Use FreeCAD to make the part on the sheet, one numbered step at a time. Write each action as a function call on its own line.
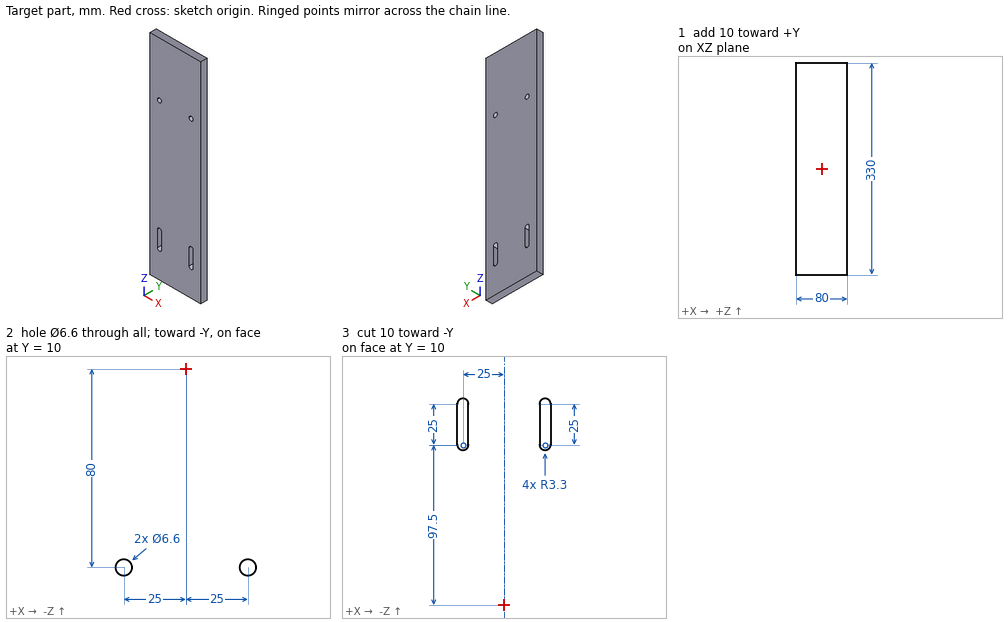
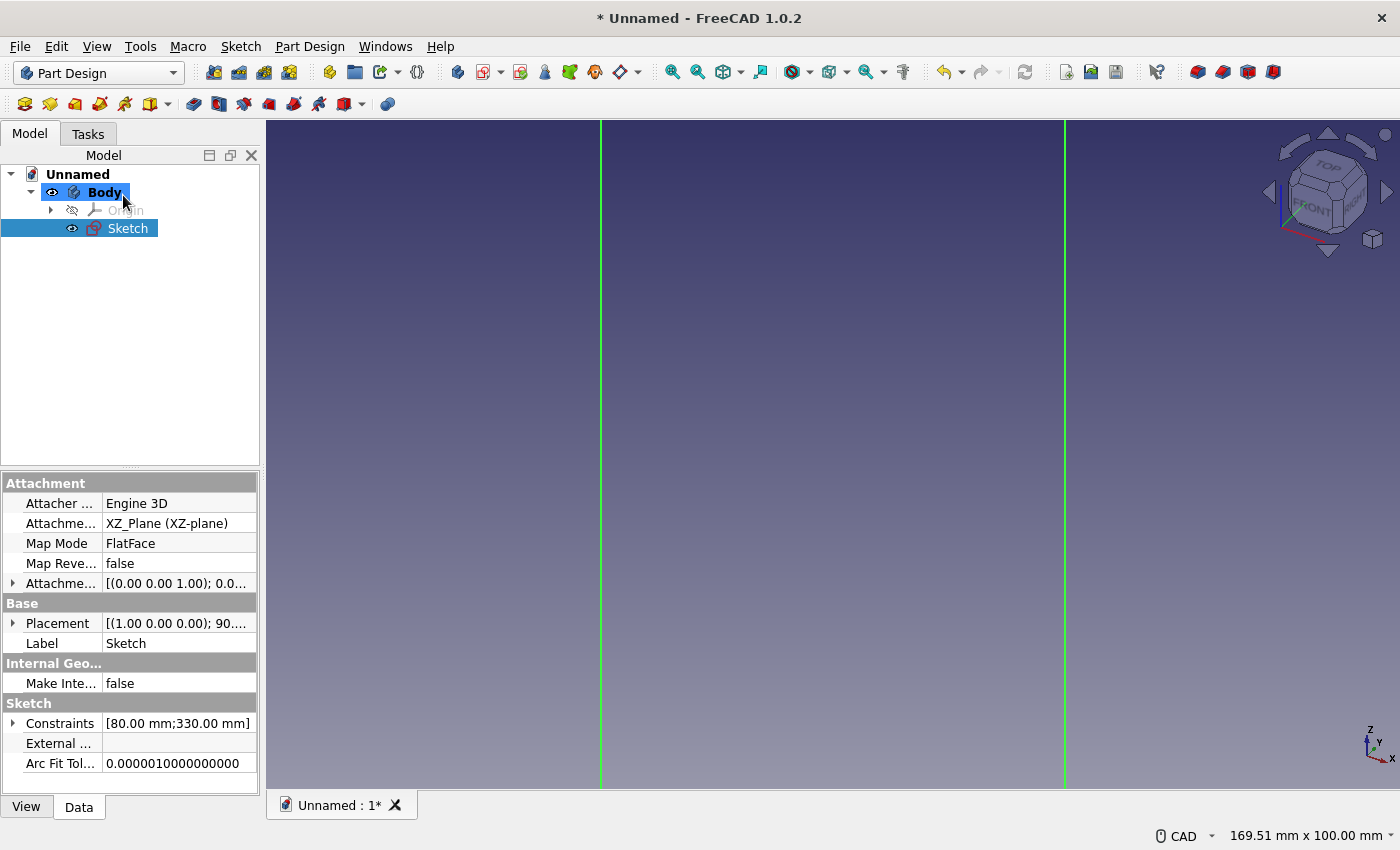
click(25, 104)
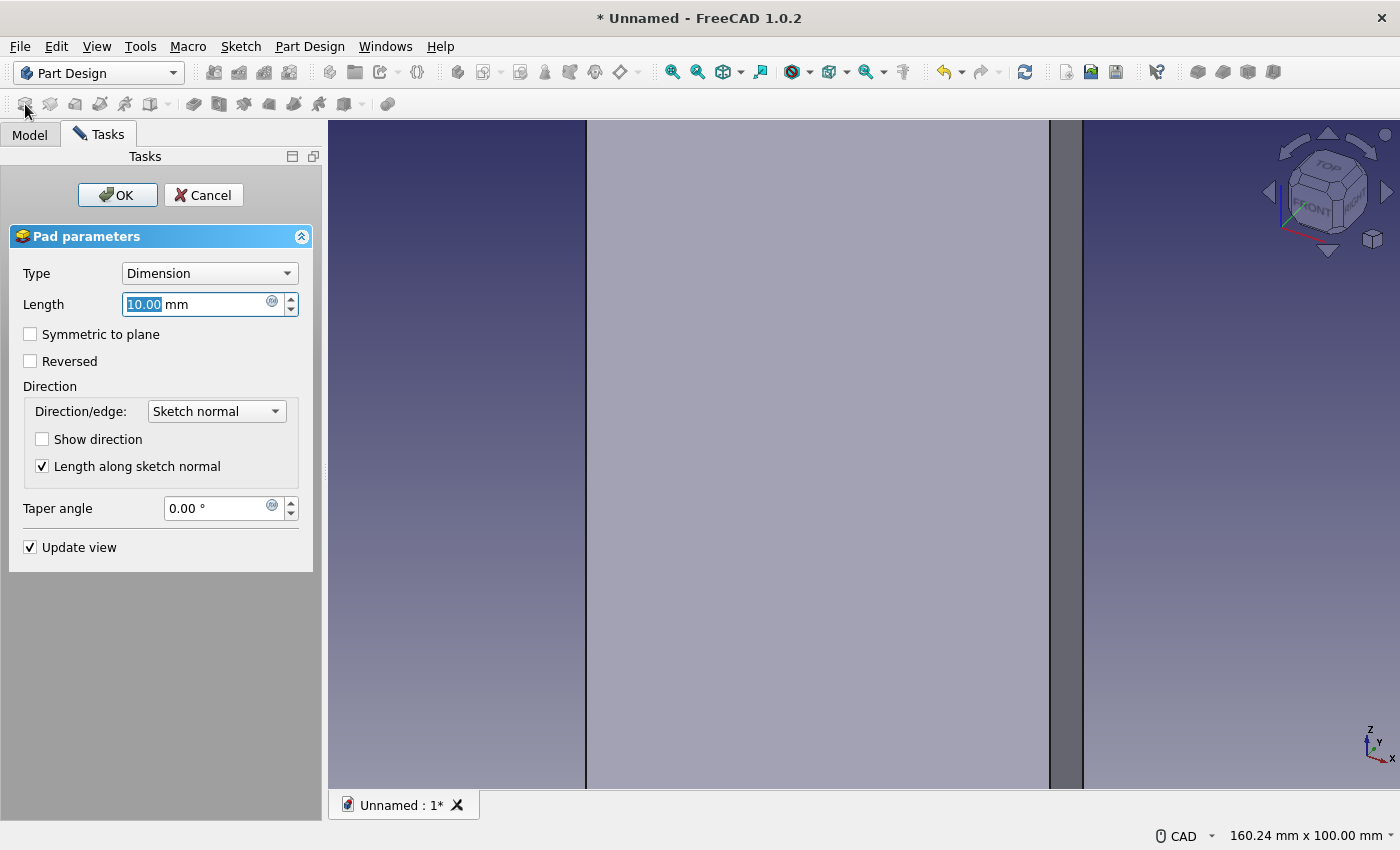
text(10)
key(Tab)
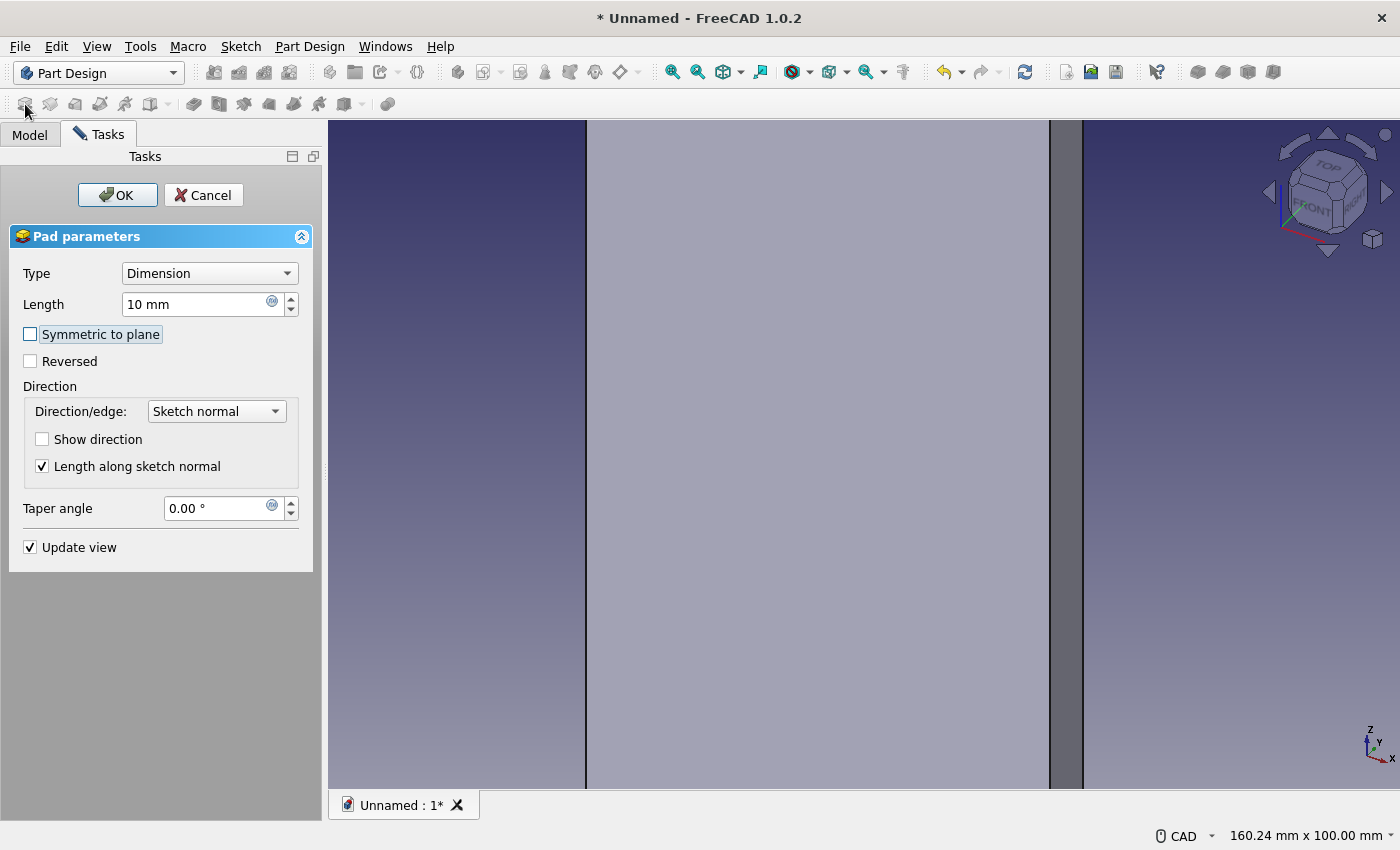
click(31, 361)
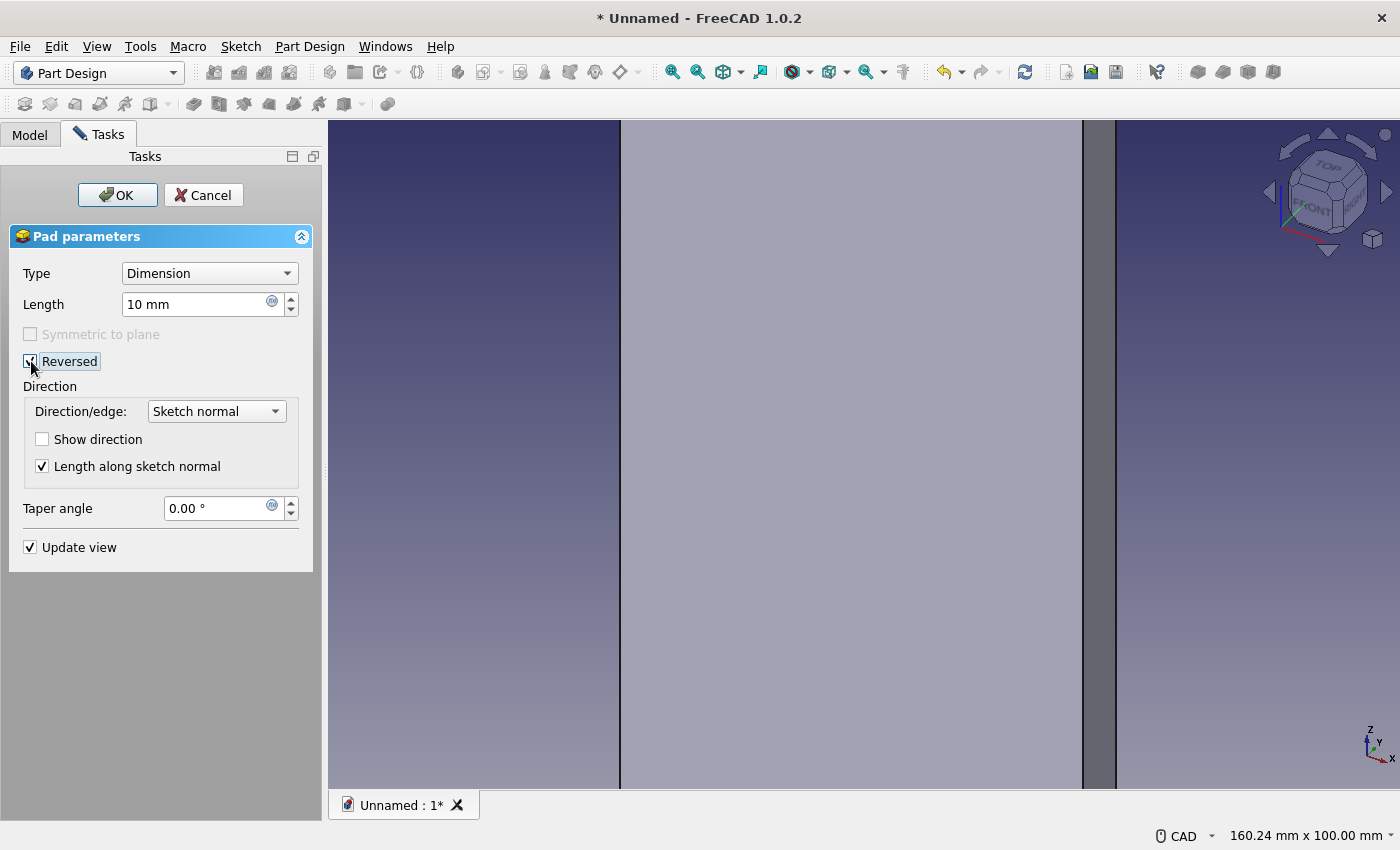
click(118, 195)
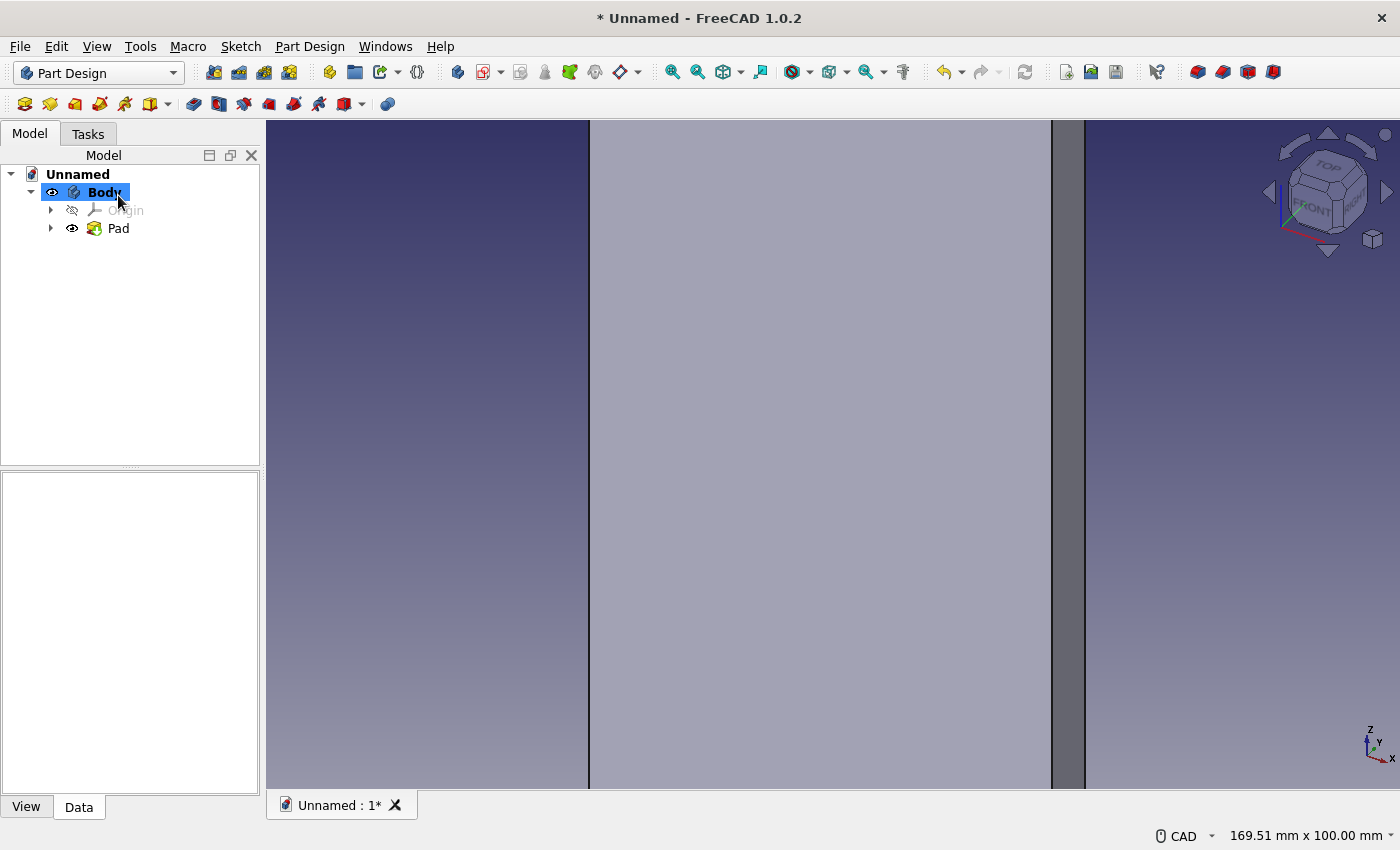
key(v)
key(f)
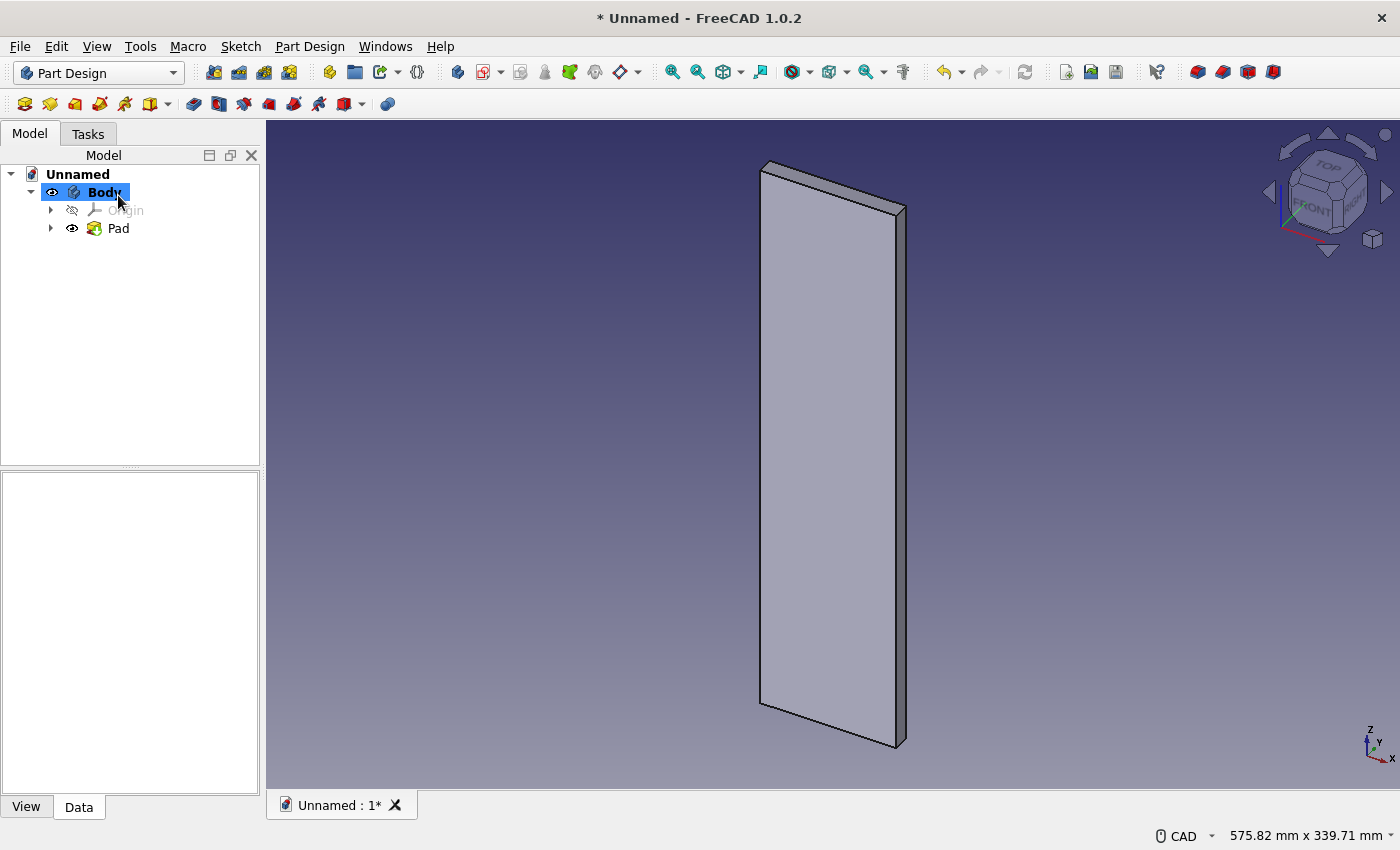
key(4)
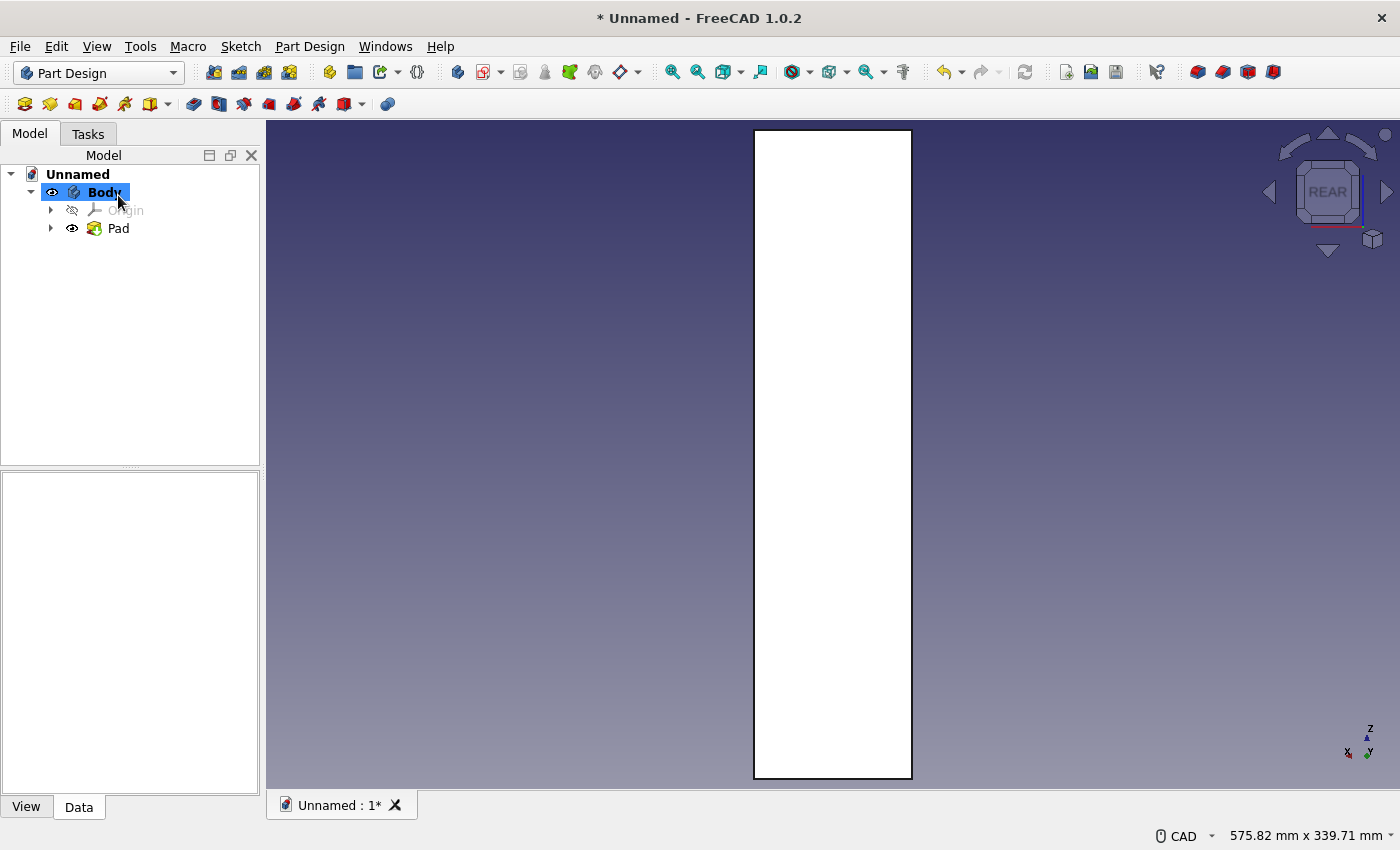
click(833, 268)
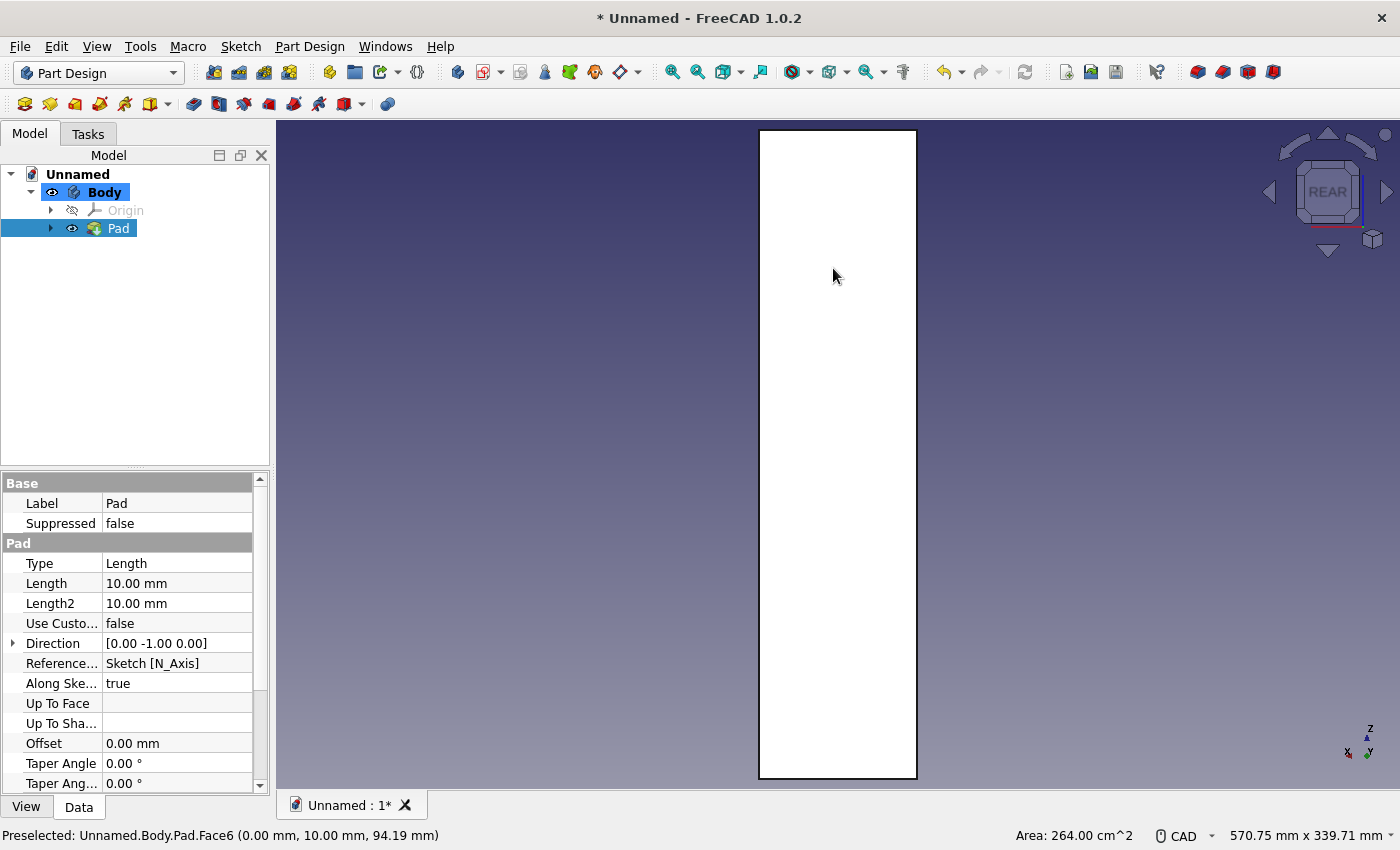
click(482, 72)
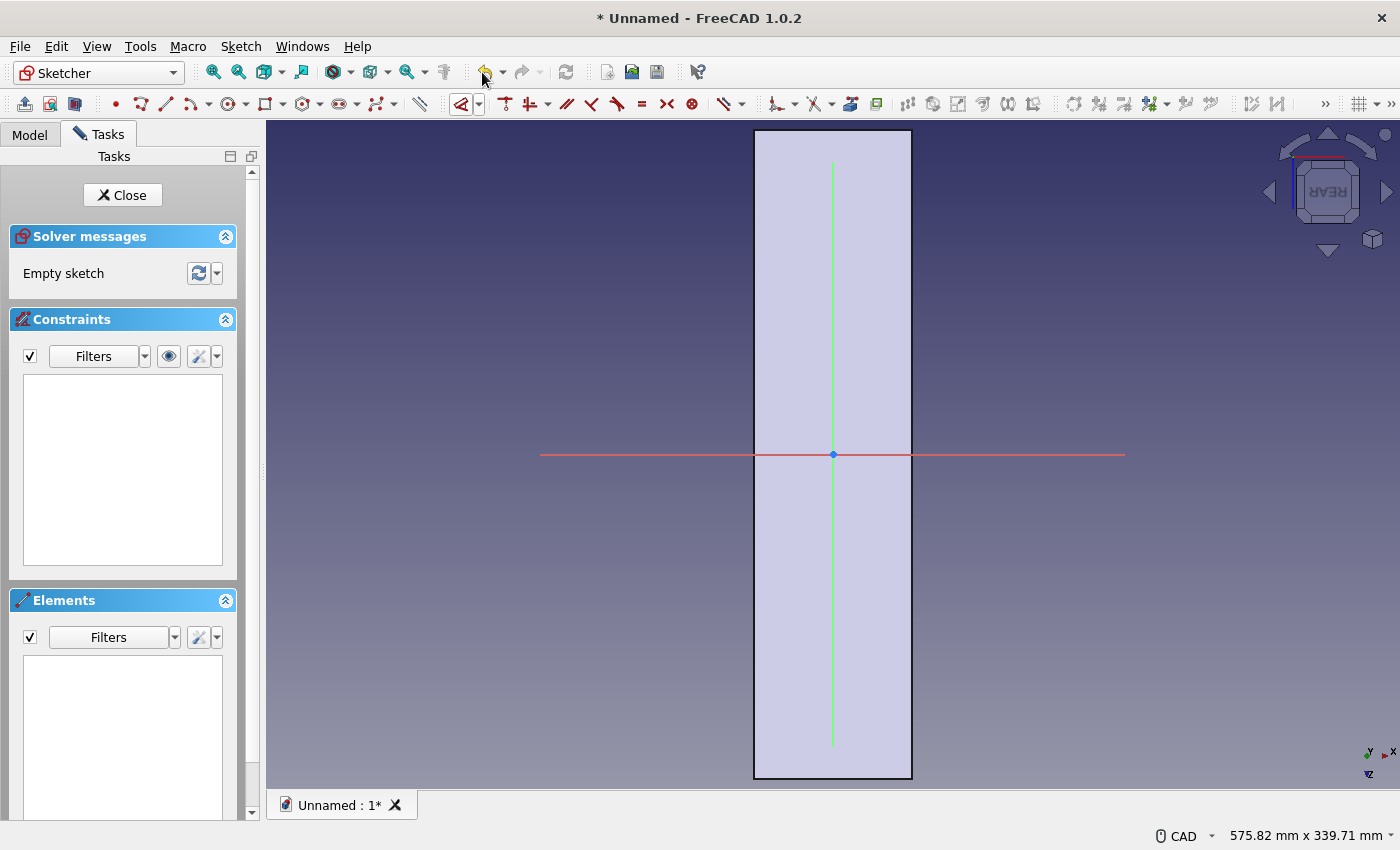
scroll(873, 584, up, 5)